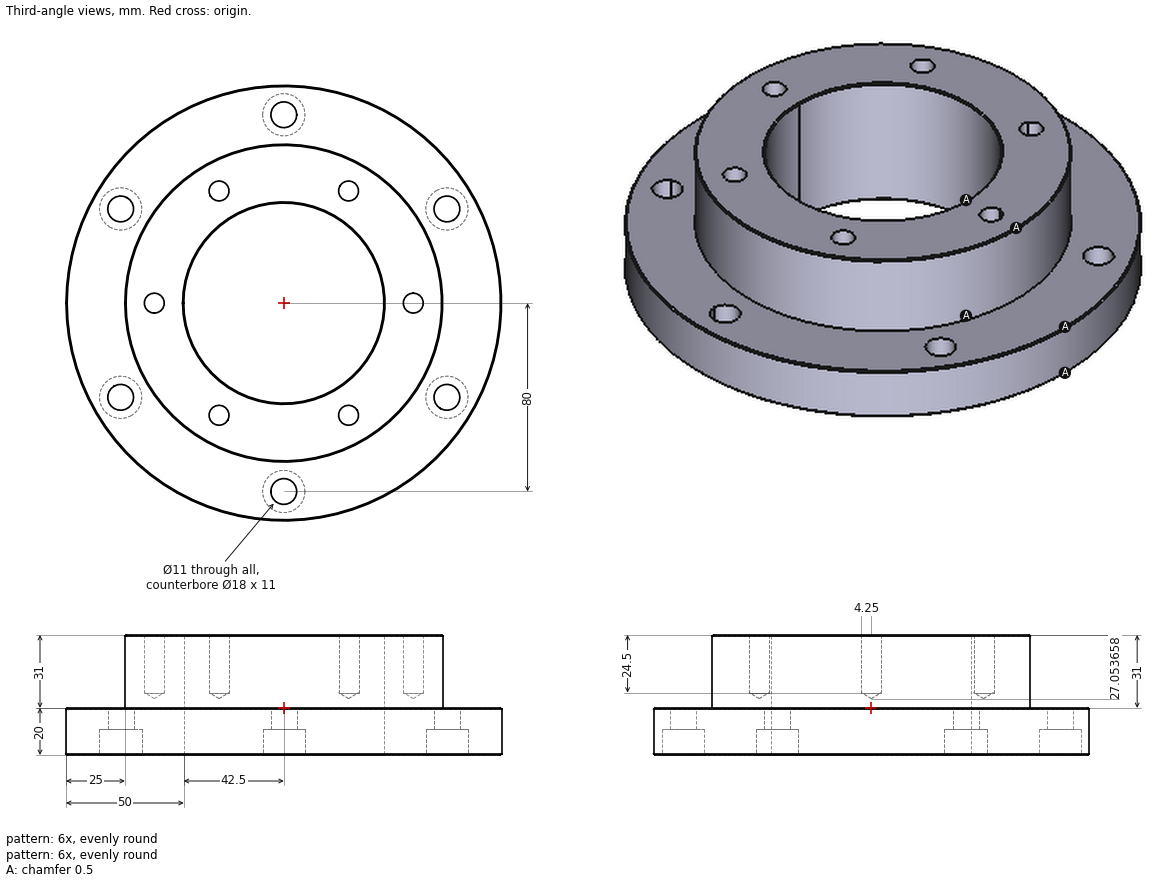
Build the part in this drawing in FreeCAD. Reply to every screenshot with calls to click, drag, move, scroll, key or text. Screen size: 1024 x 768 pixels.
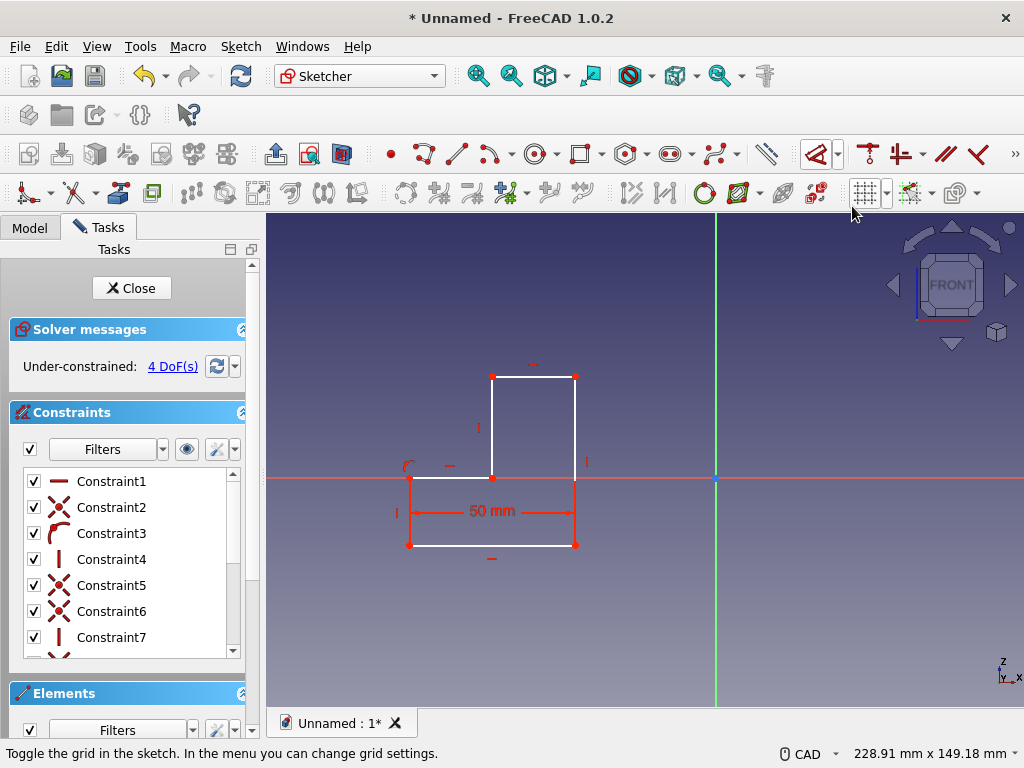
click(410, 526)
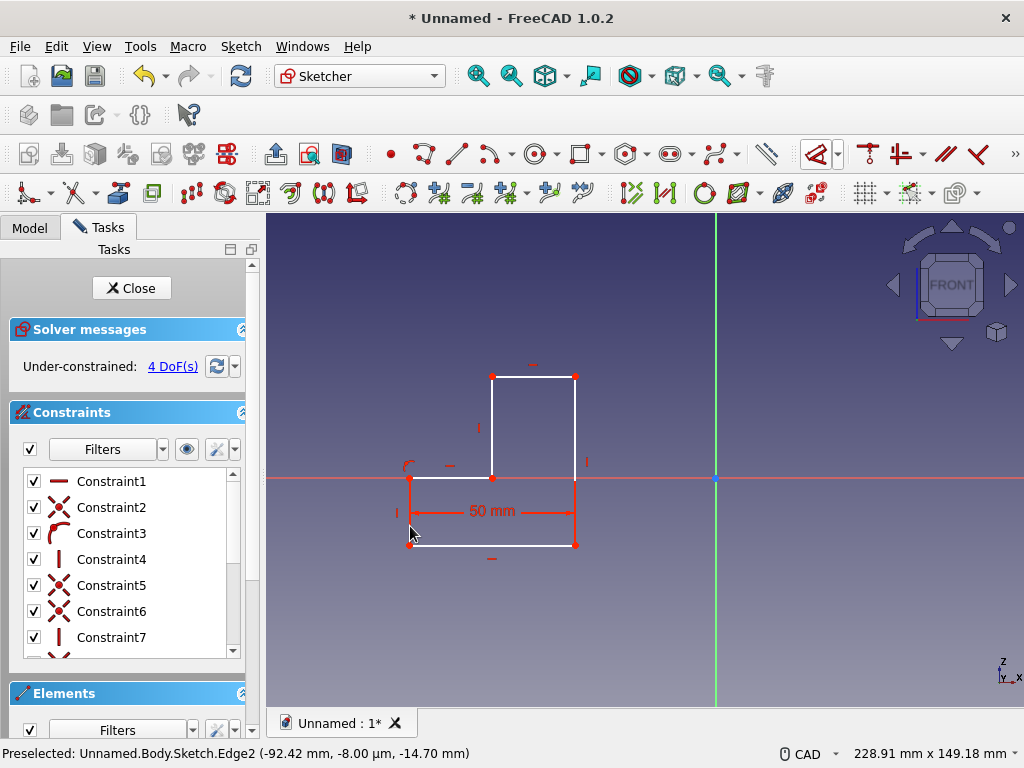
click(838, 154)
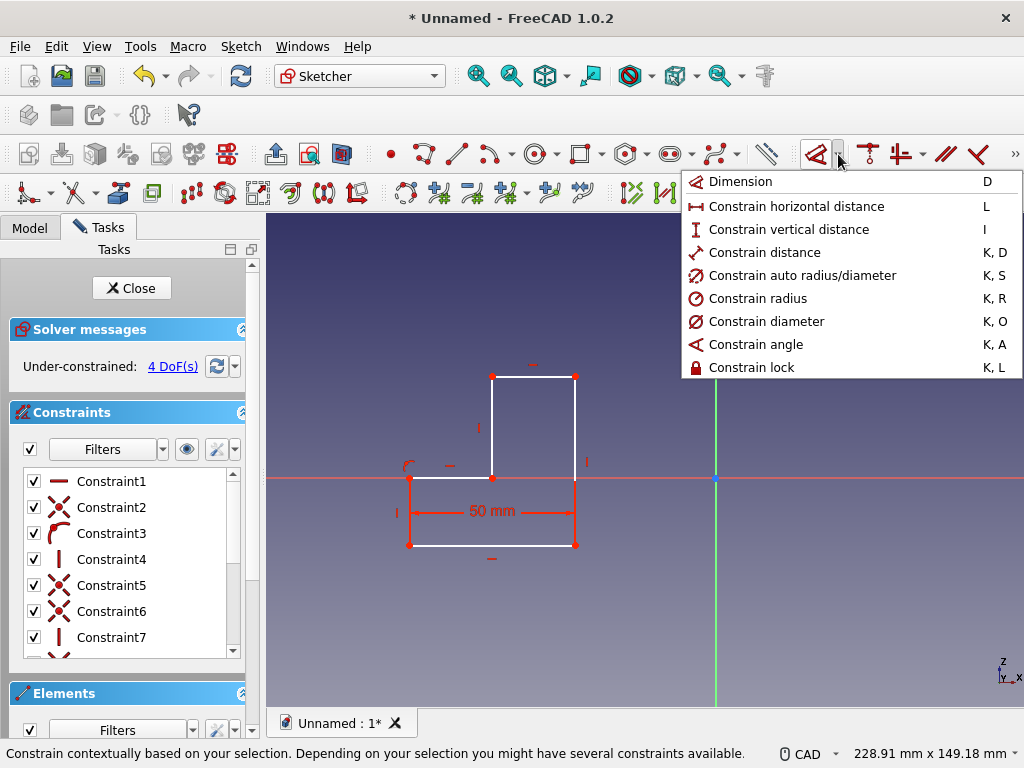
click(852, 230)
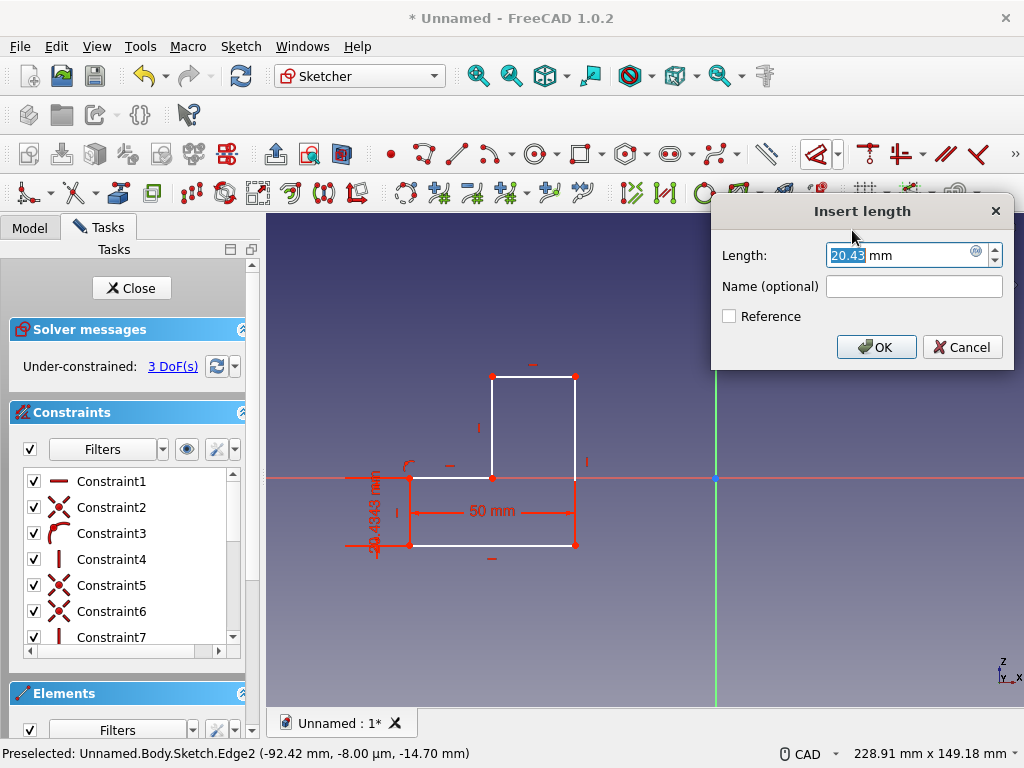
text(20)
key(Return)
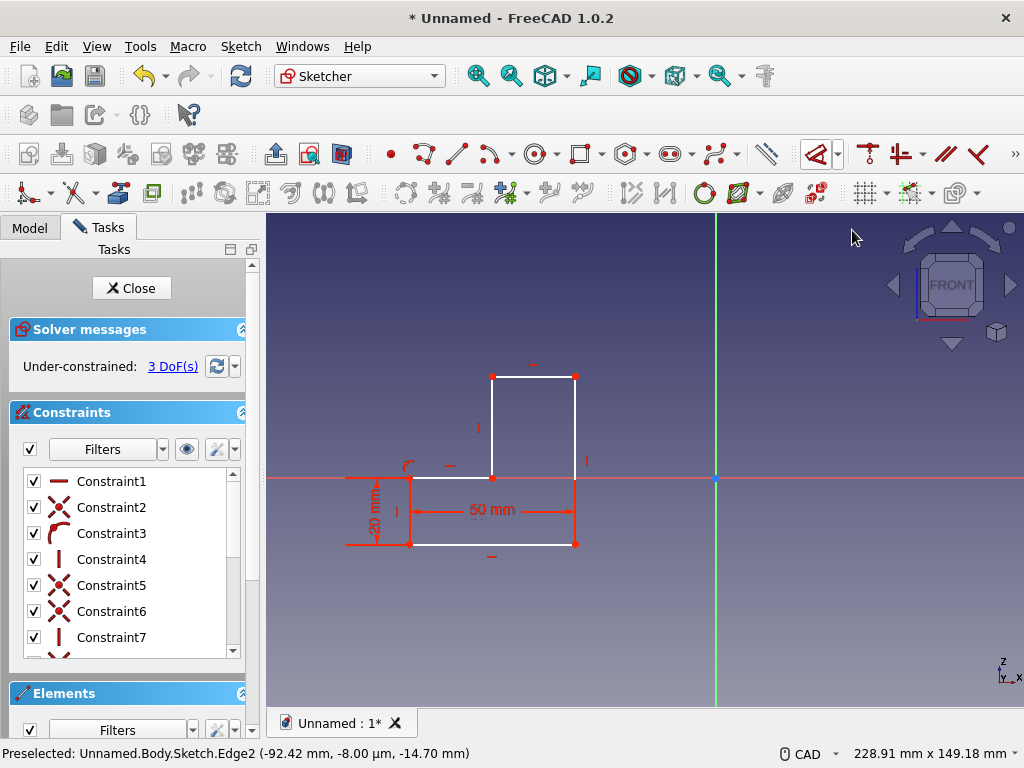
click(434, 478)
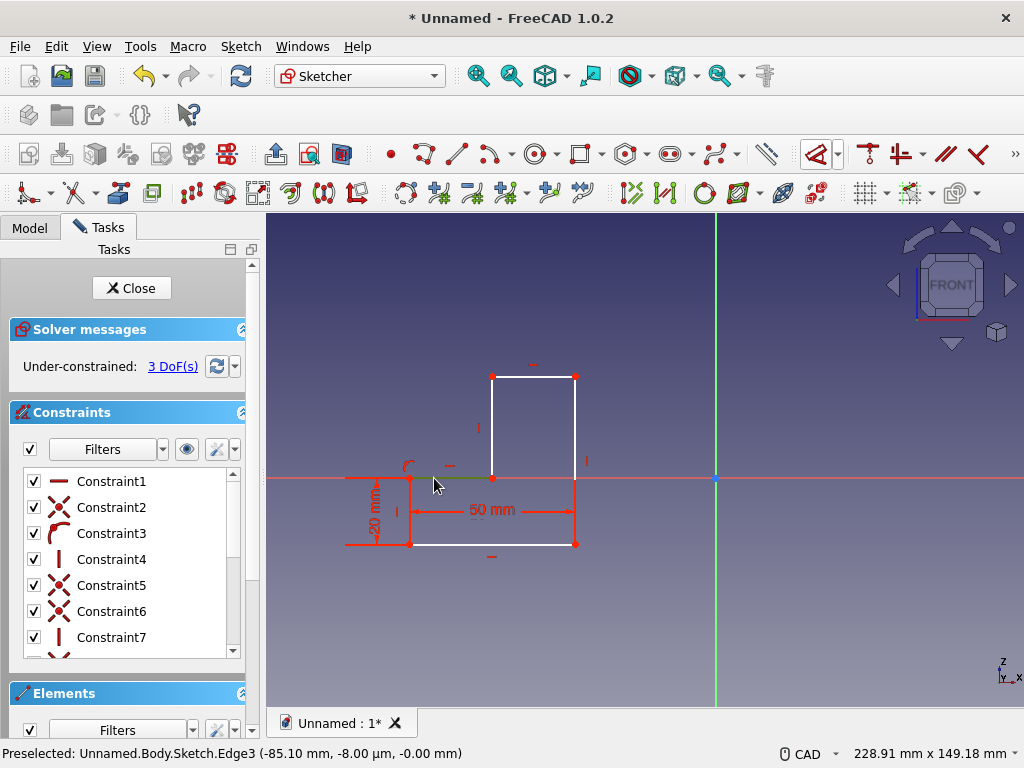
click(838, 154)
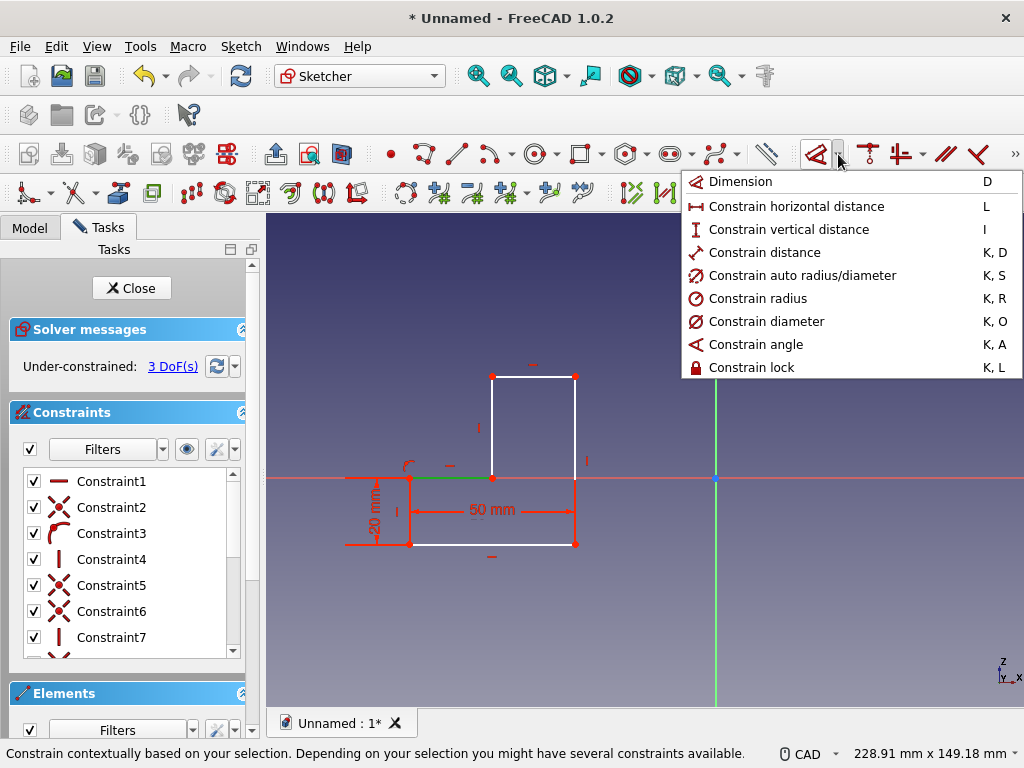
click(852, 206)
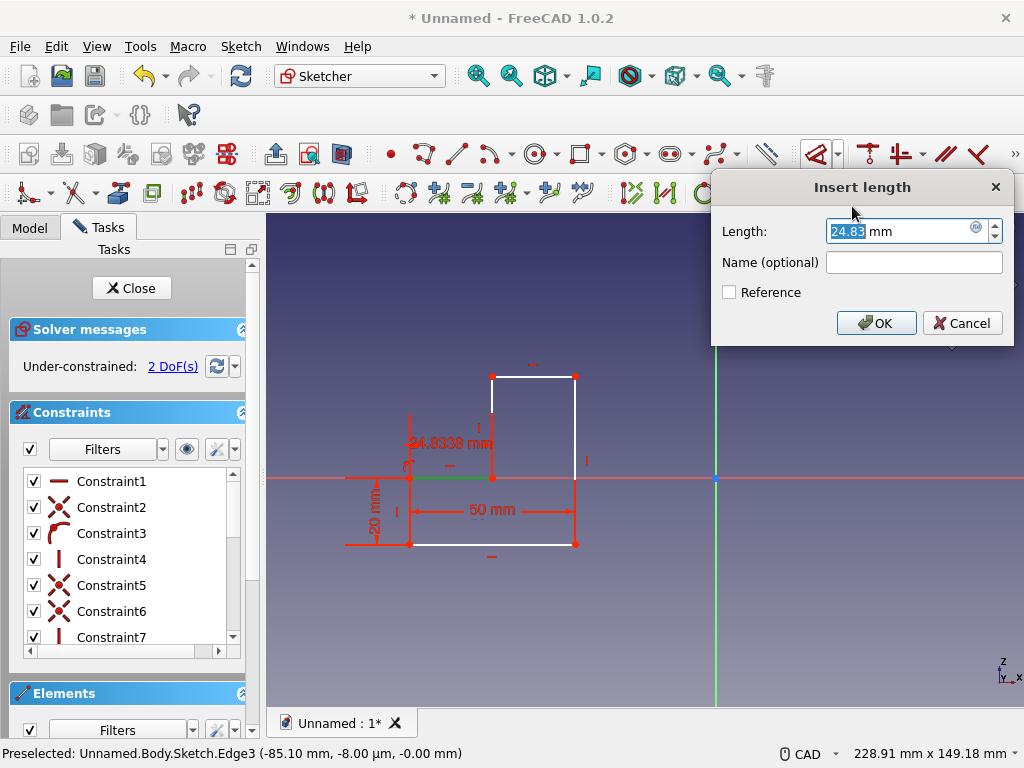
text(25)
key(Return)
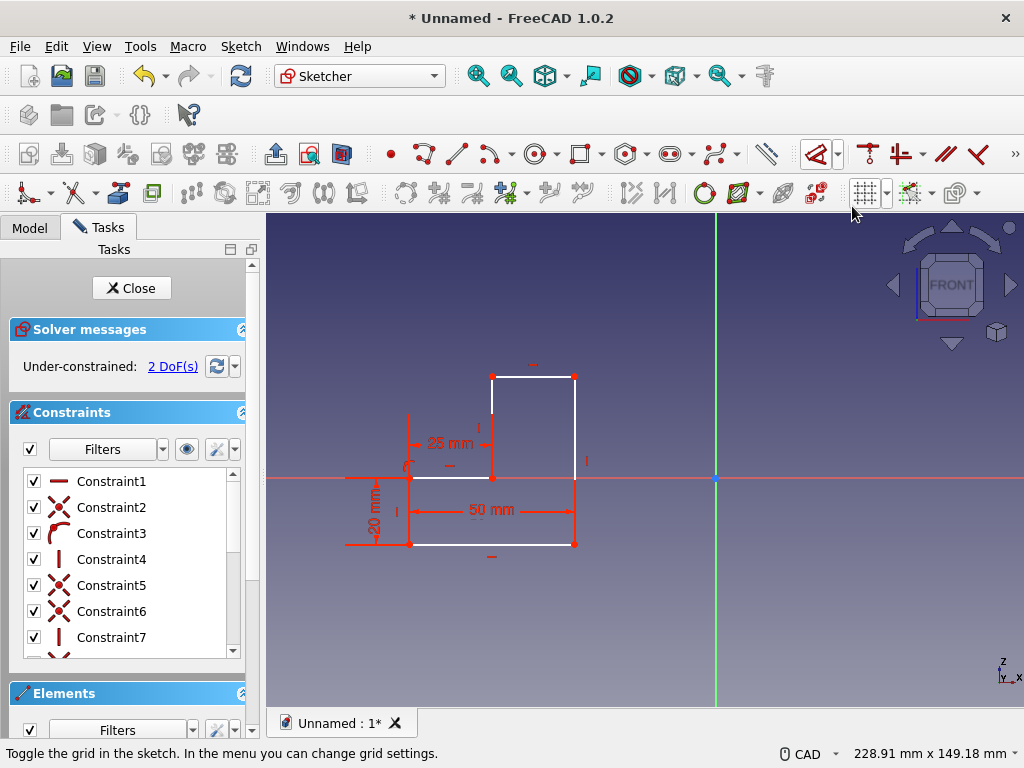
click(492, 448)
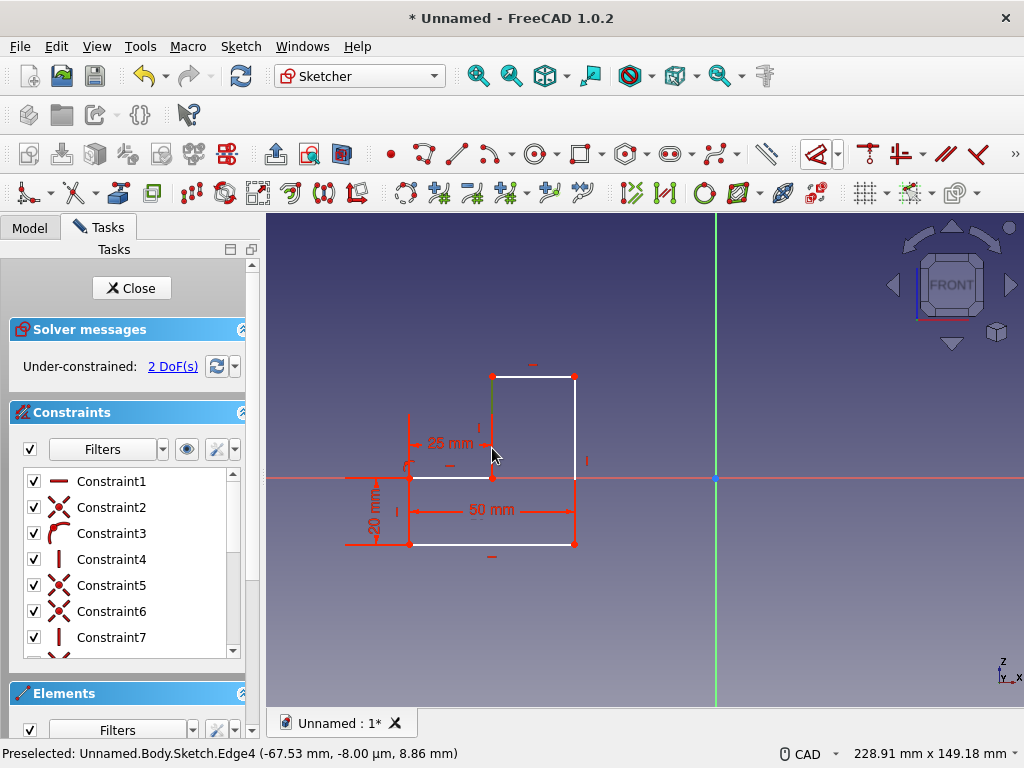
click(838, 154)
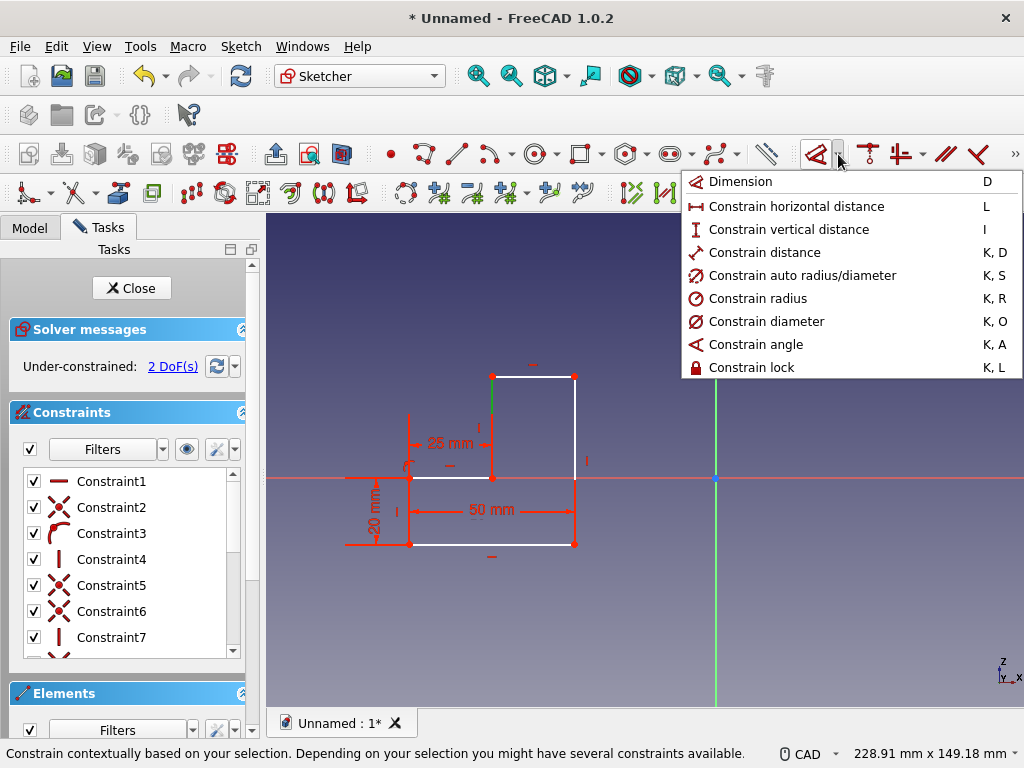
click(852, 230)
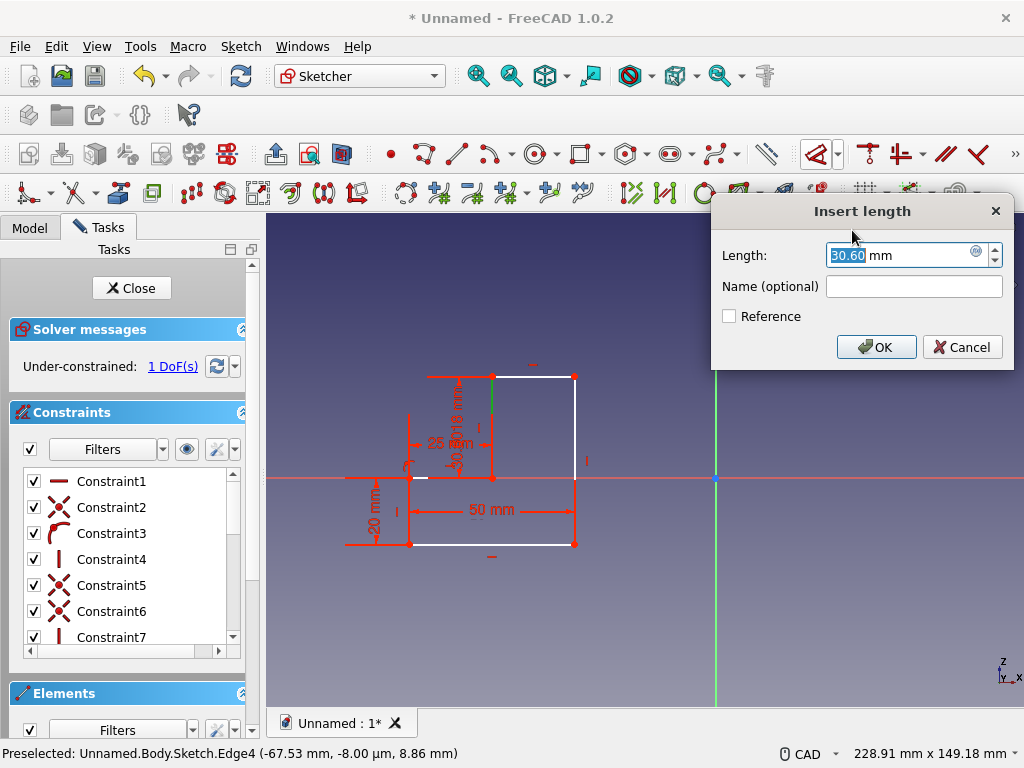
text(31)
key(Return)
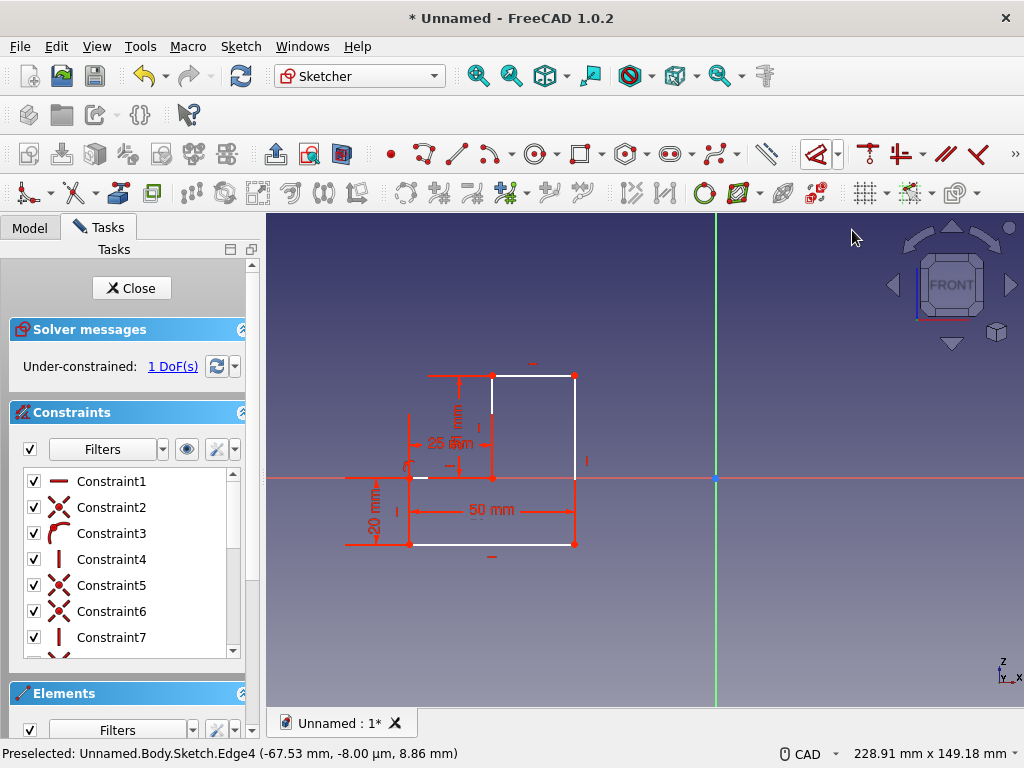
click(575, 545)